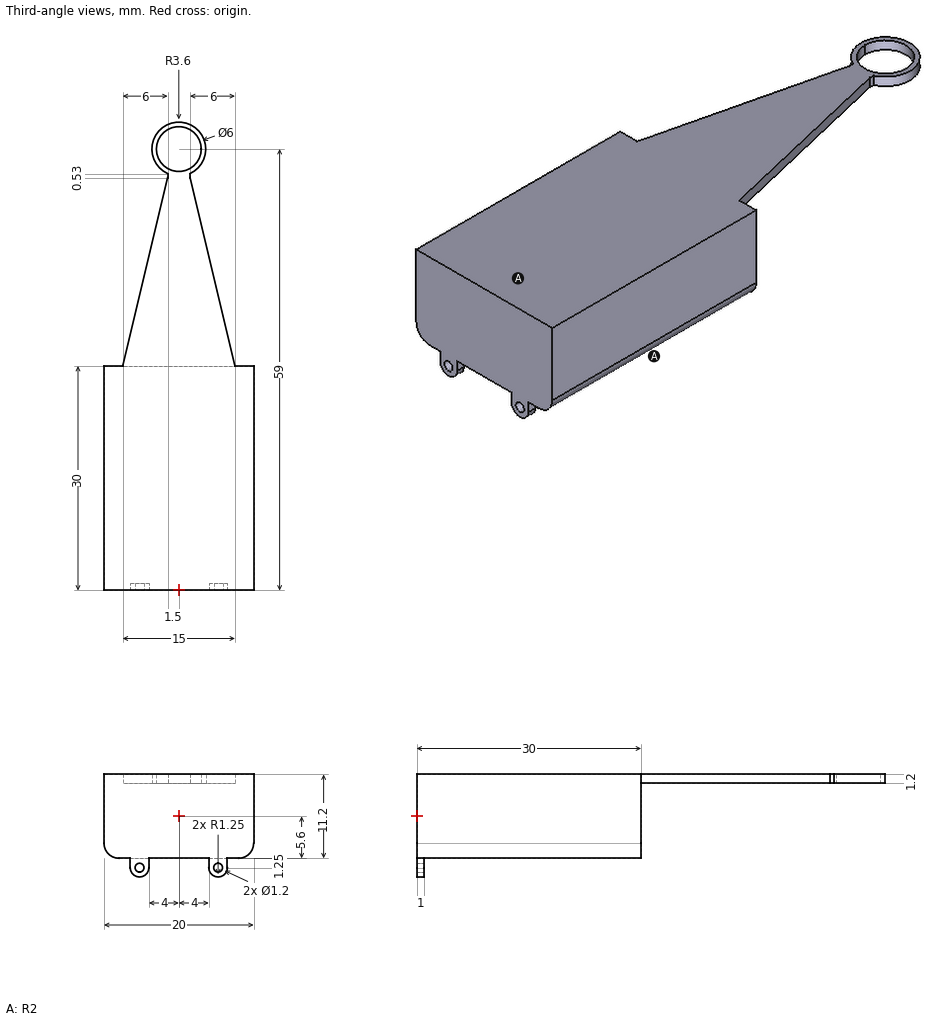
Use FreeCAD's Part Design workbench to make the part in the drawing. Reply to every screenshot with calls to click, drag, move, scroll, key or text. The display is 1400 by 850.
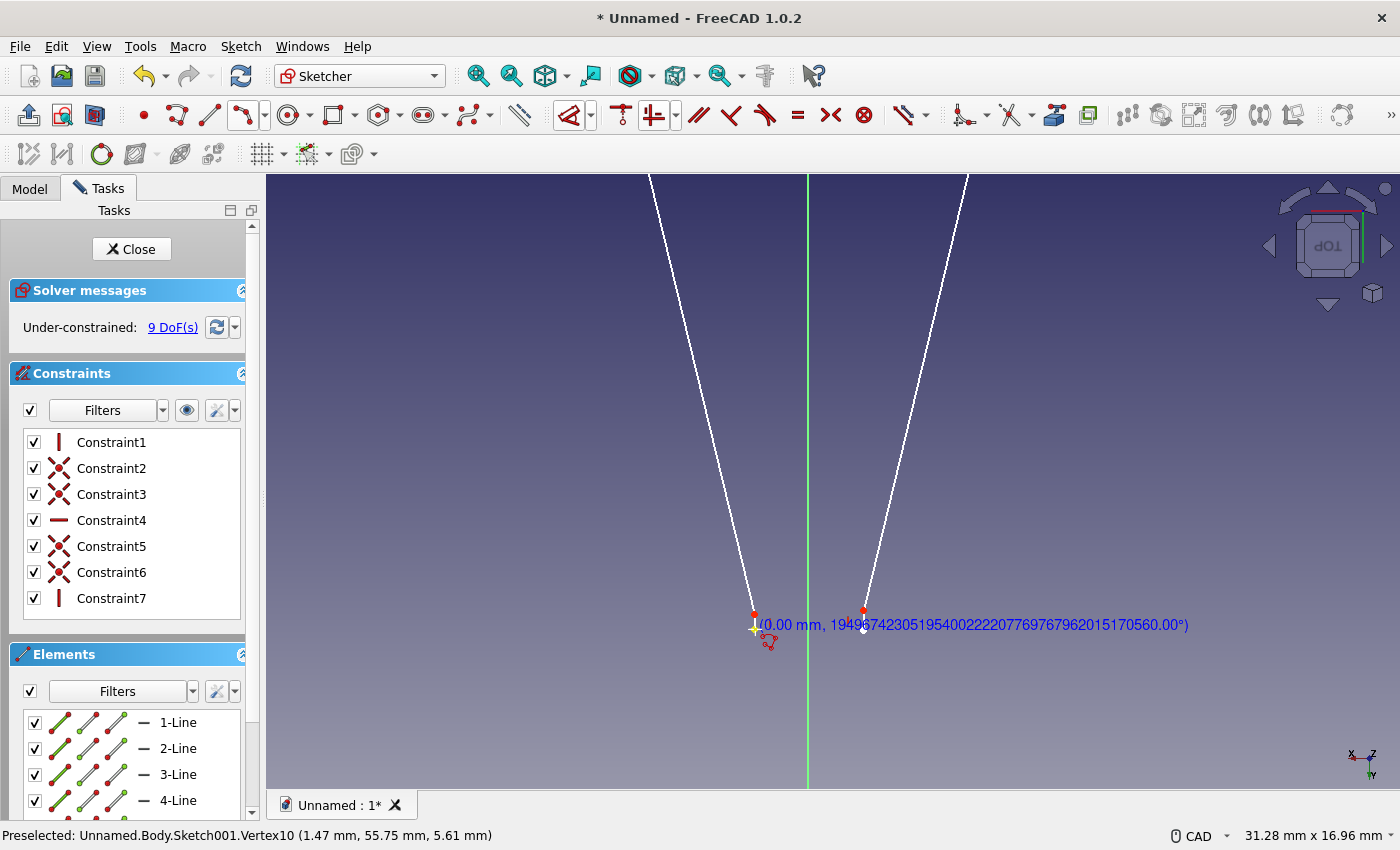
click(242, 116)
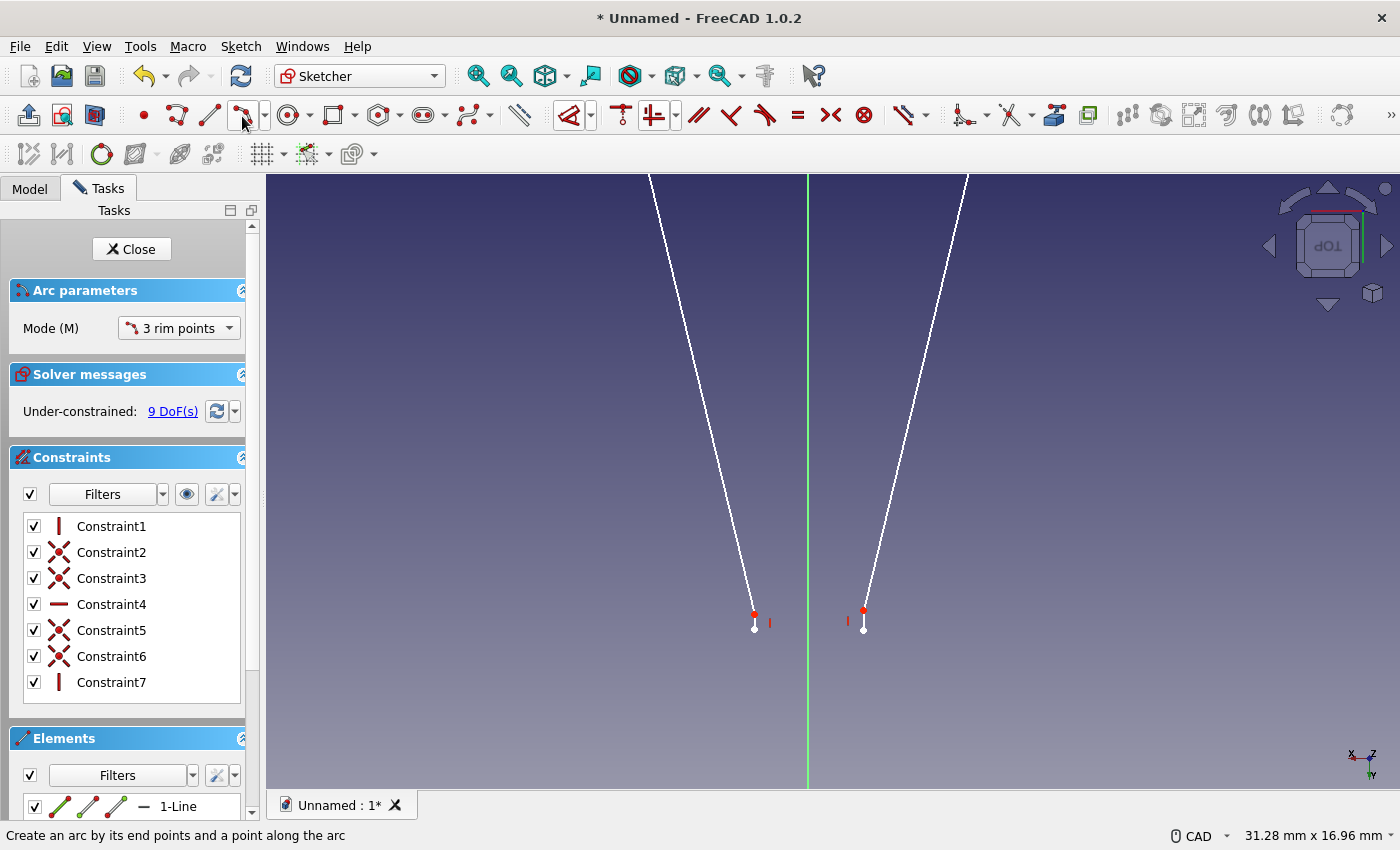
scroll(754, 629, up, 3)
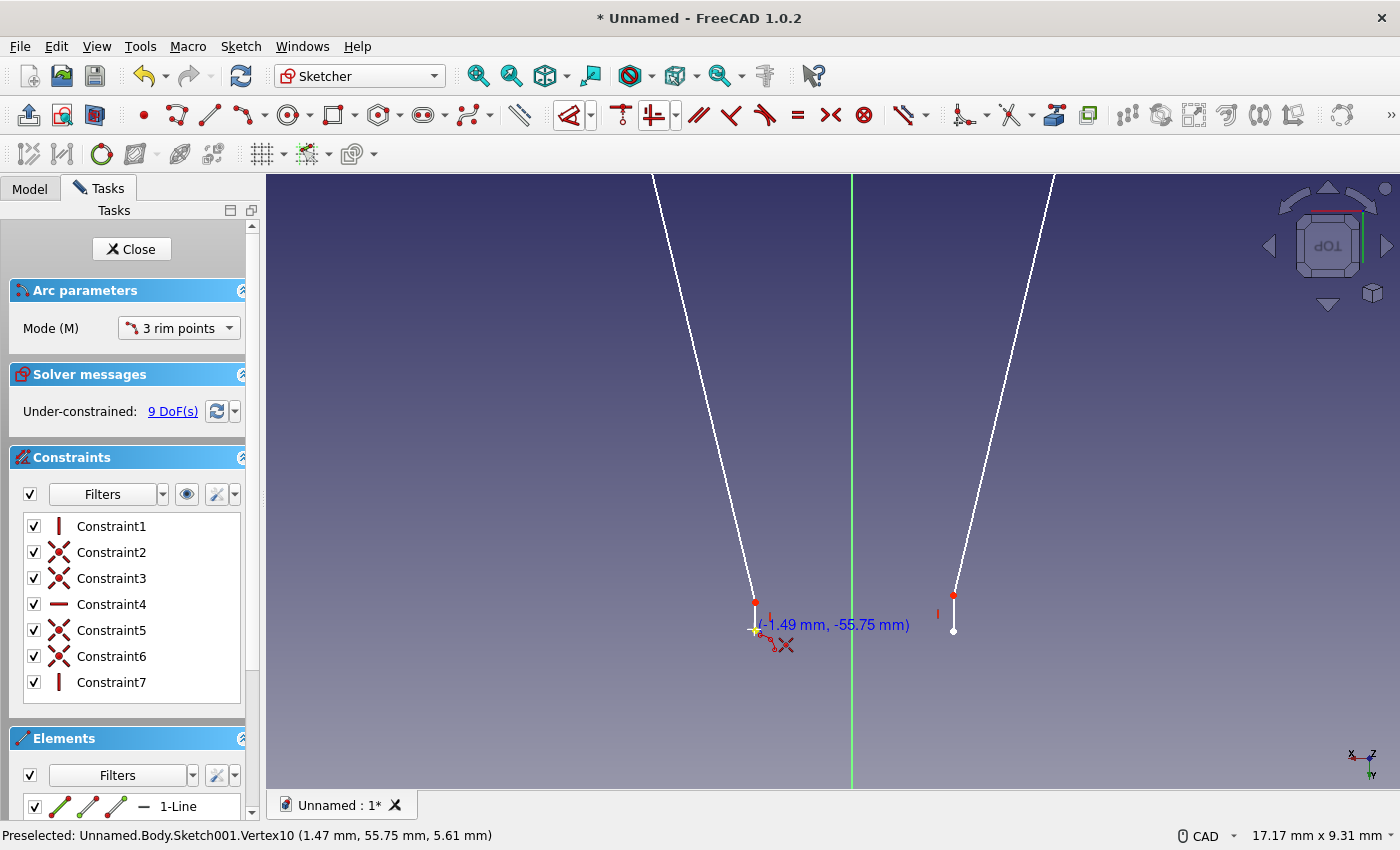
click(755, 630)
click(954, 632)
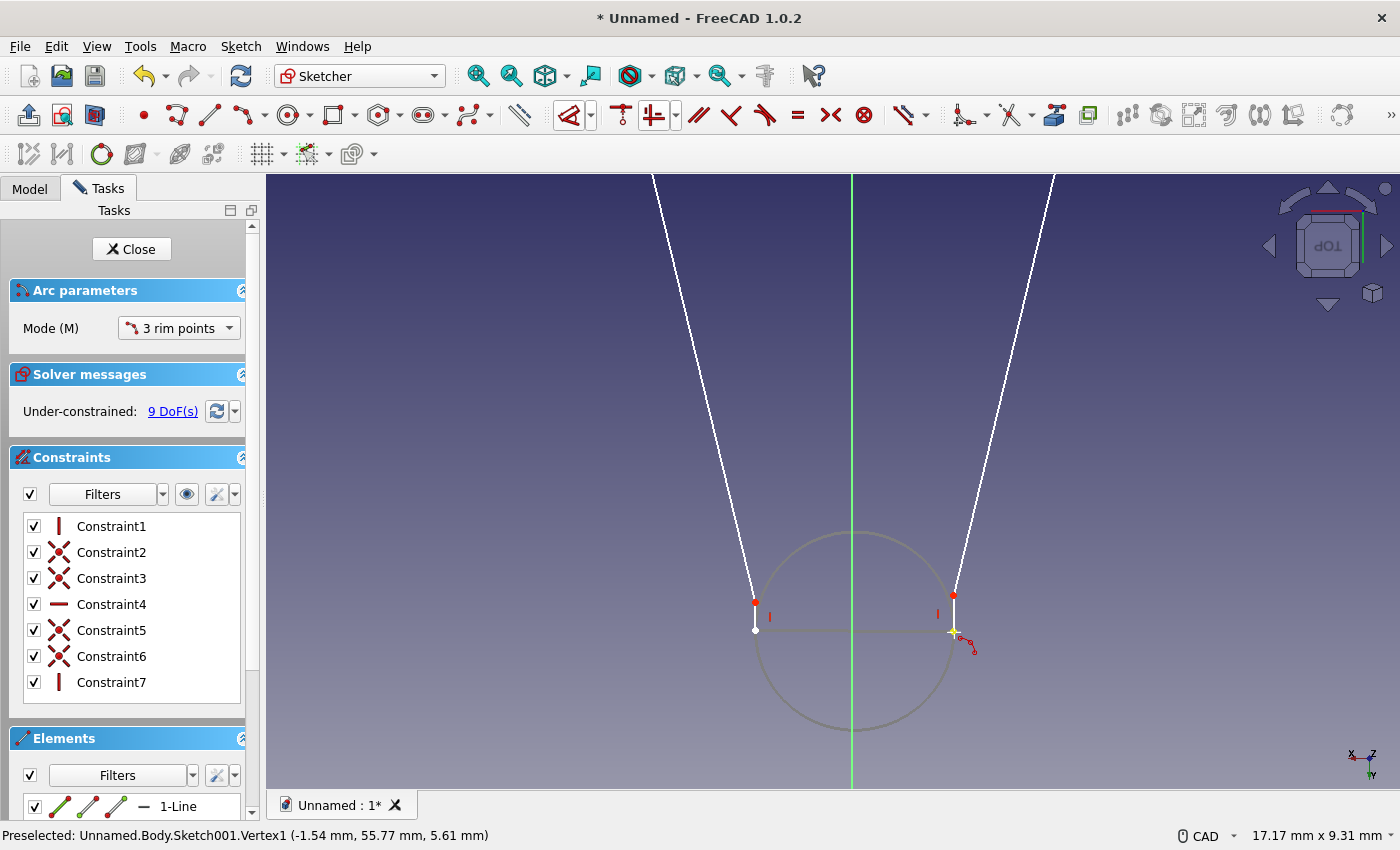
scroll(756, 628, down, 12)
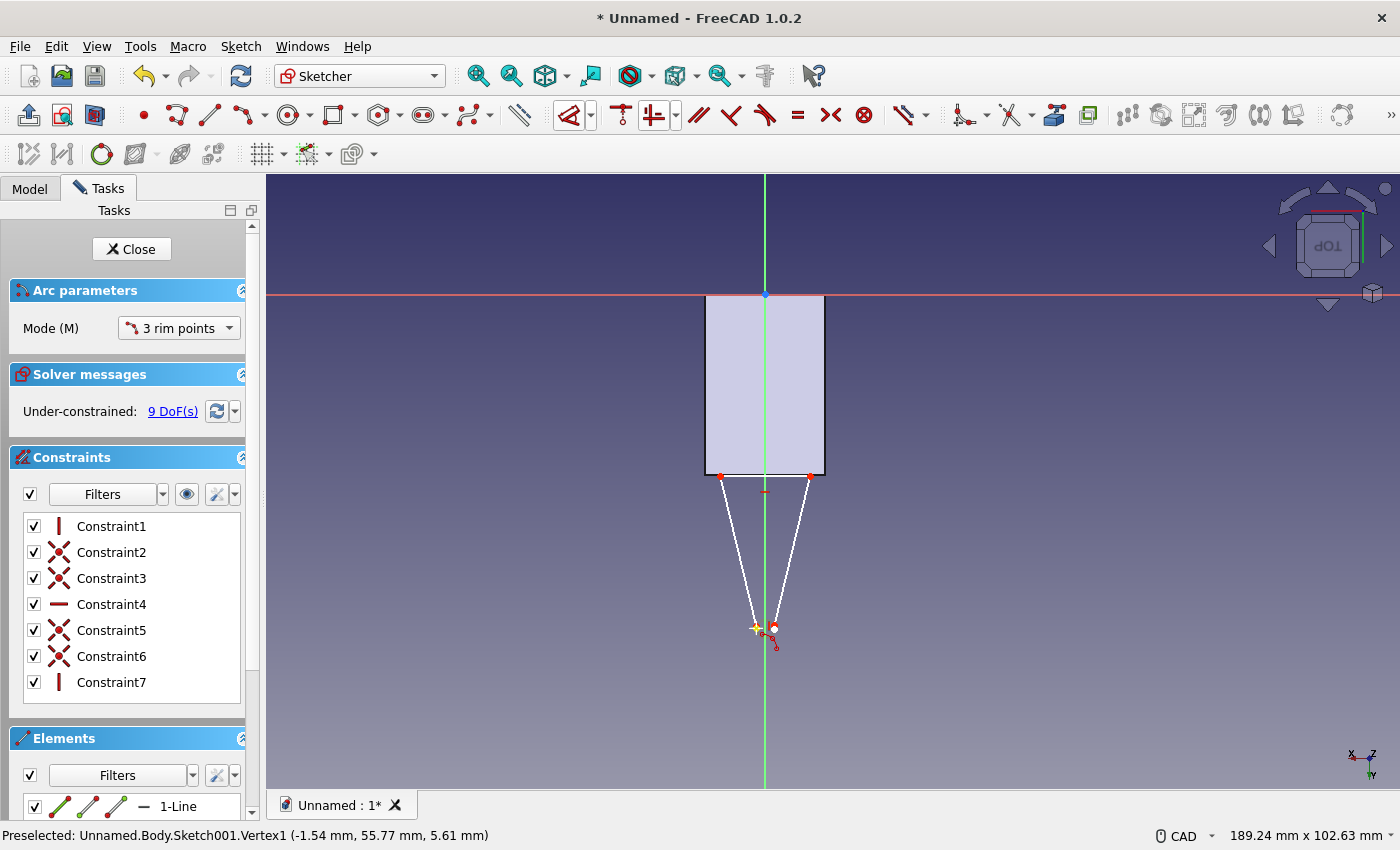
click(746, 658)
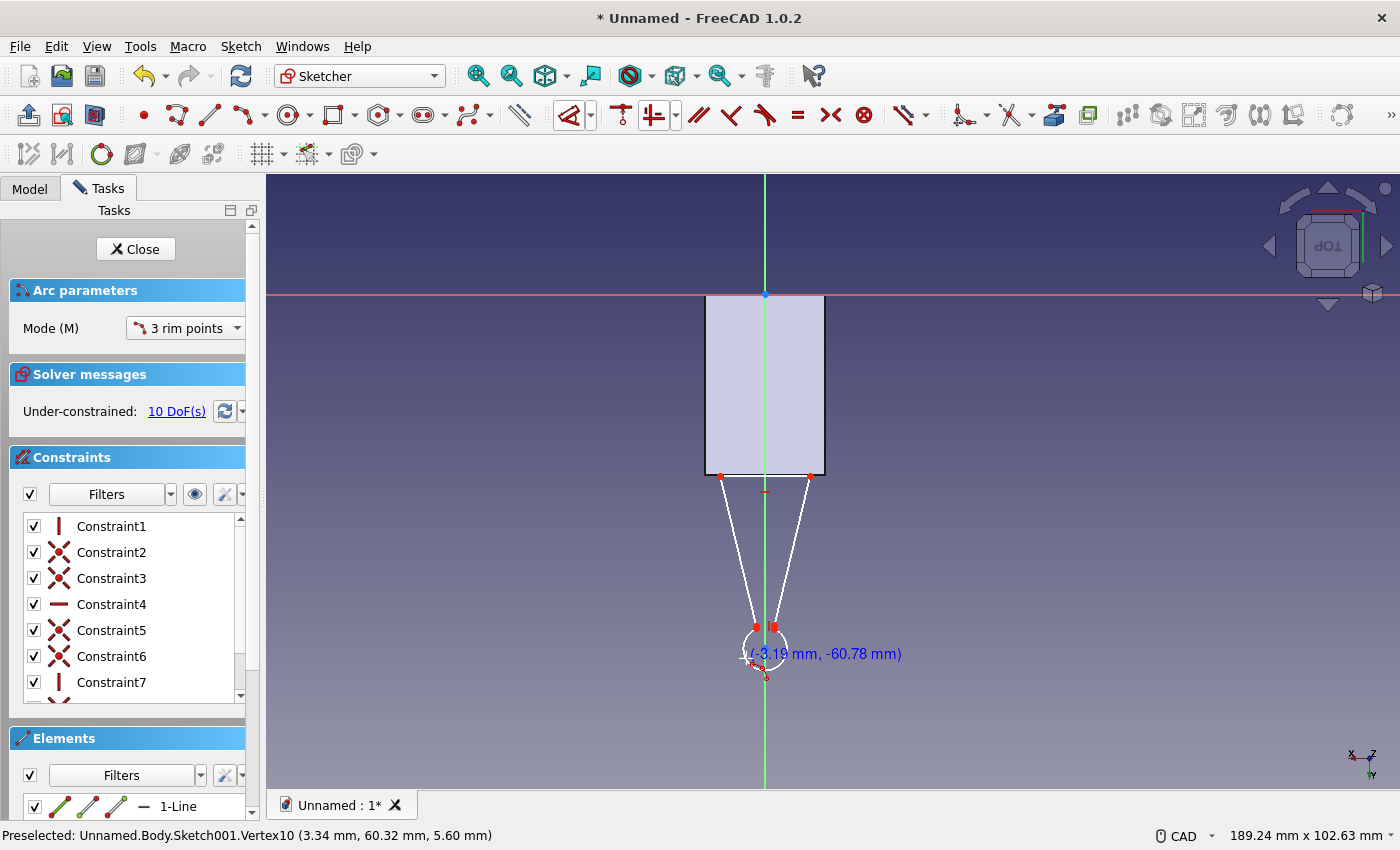
key(g)
key(c)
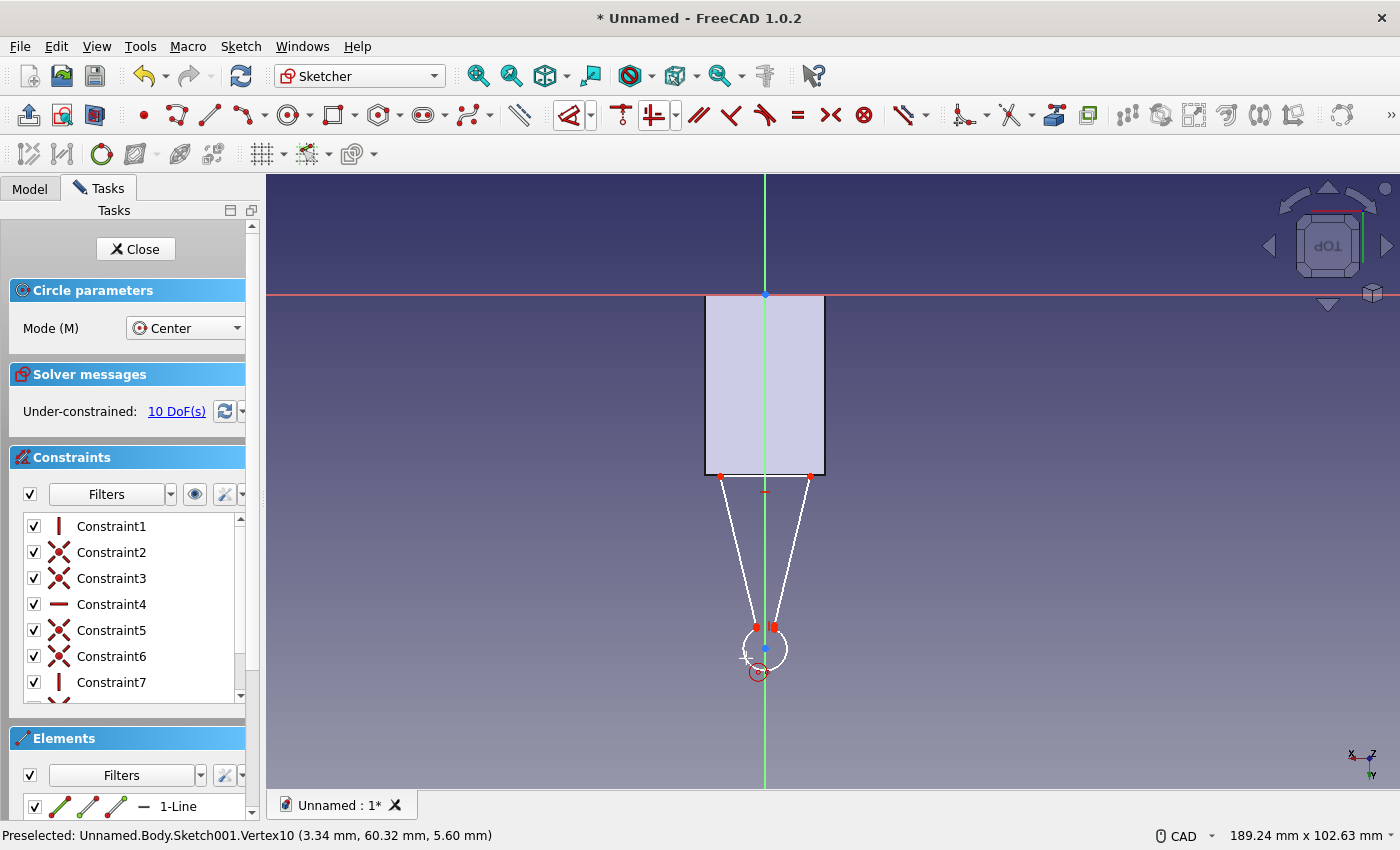
scroll(765, 648, up, 2)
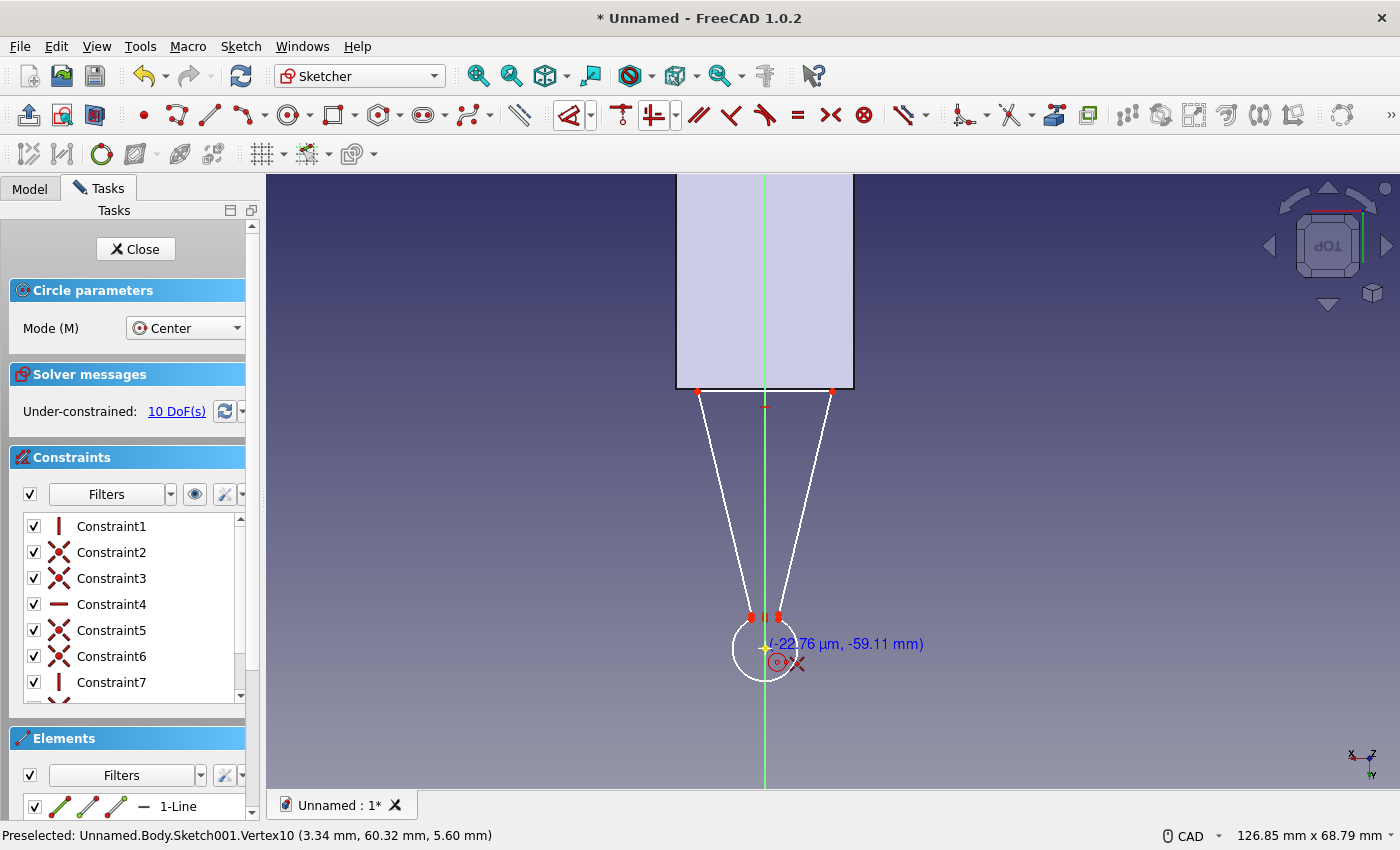
click(765, 648)